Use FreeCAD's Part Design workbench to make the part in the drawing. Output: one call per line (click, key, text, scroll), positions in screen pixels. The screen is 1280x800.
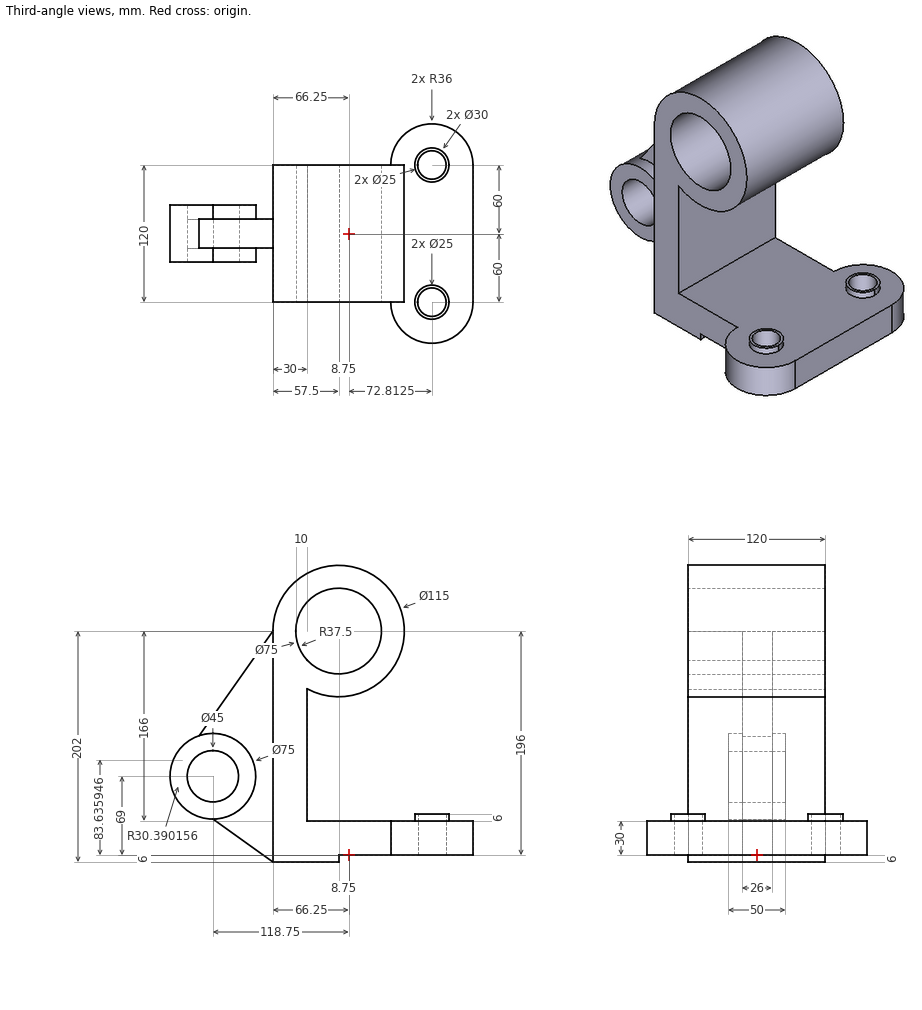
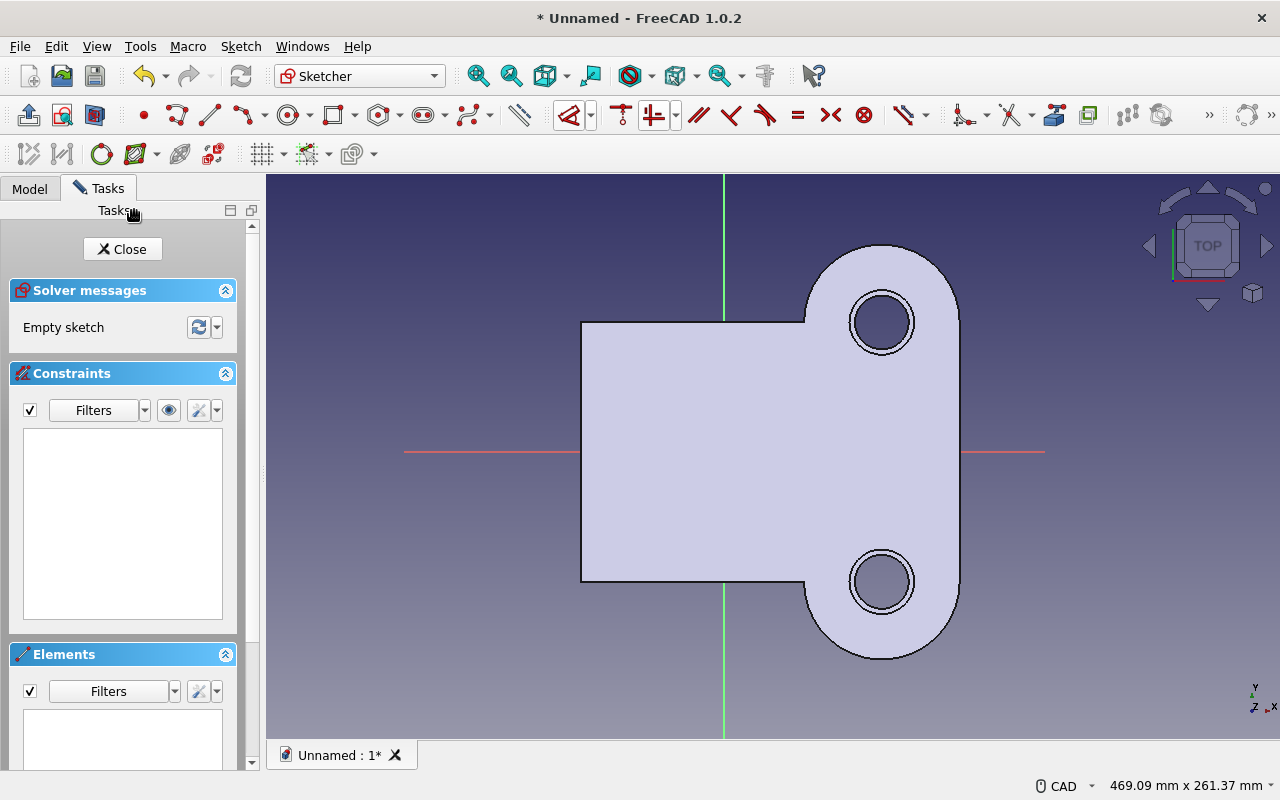
key(q)
key(s)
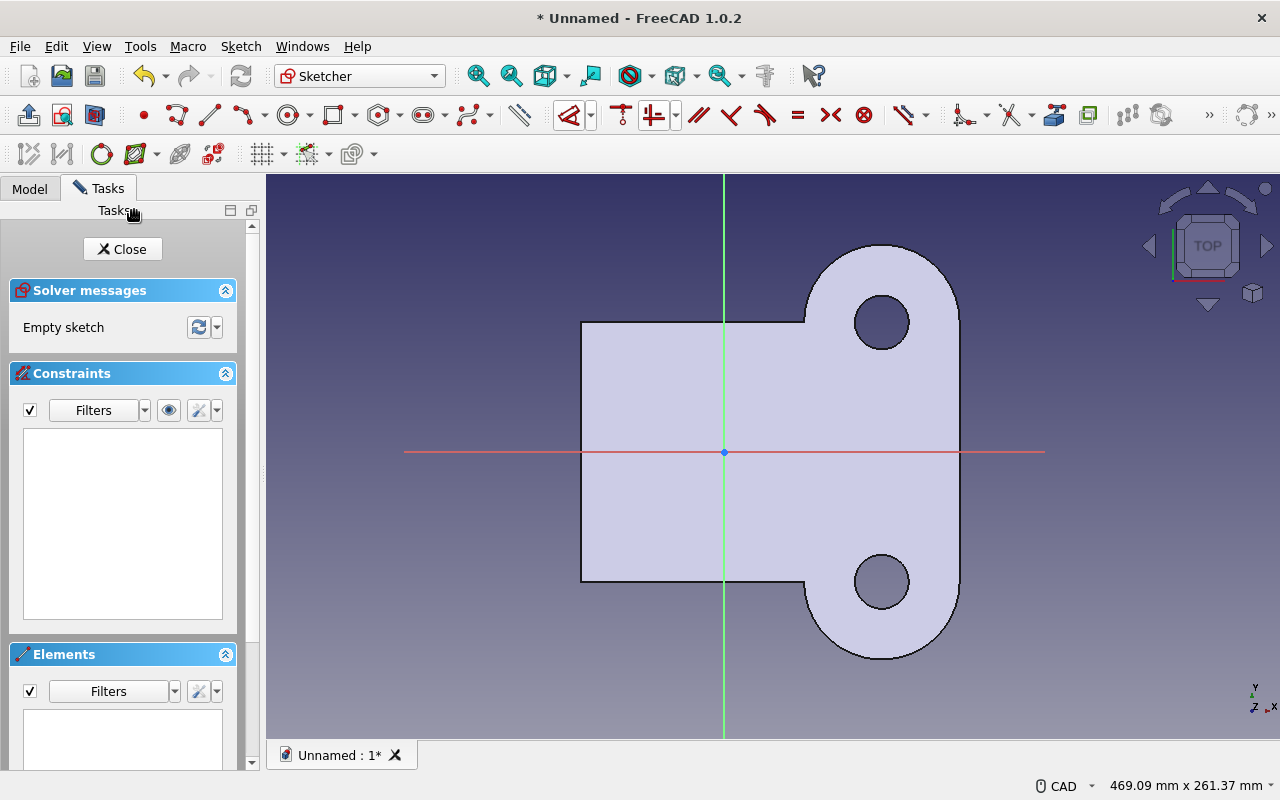
scroll(548, 443, up, 2)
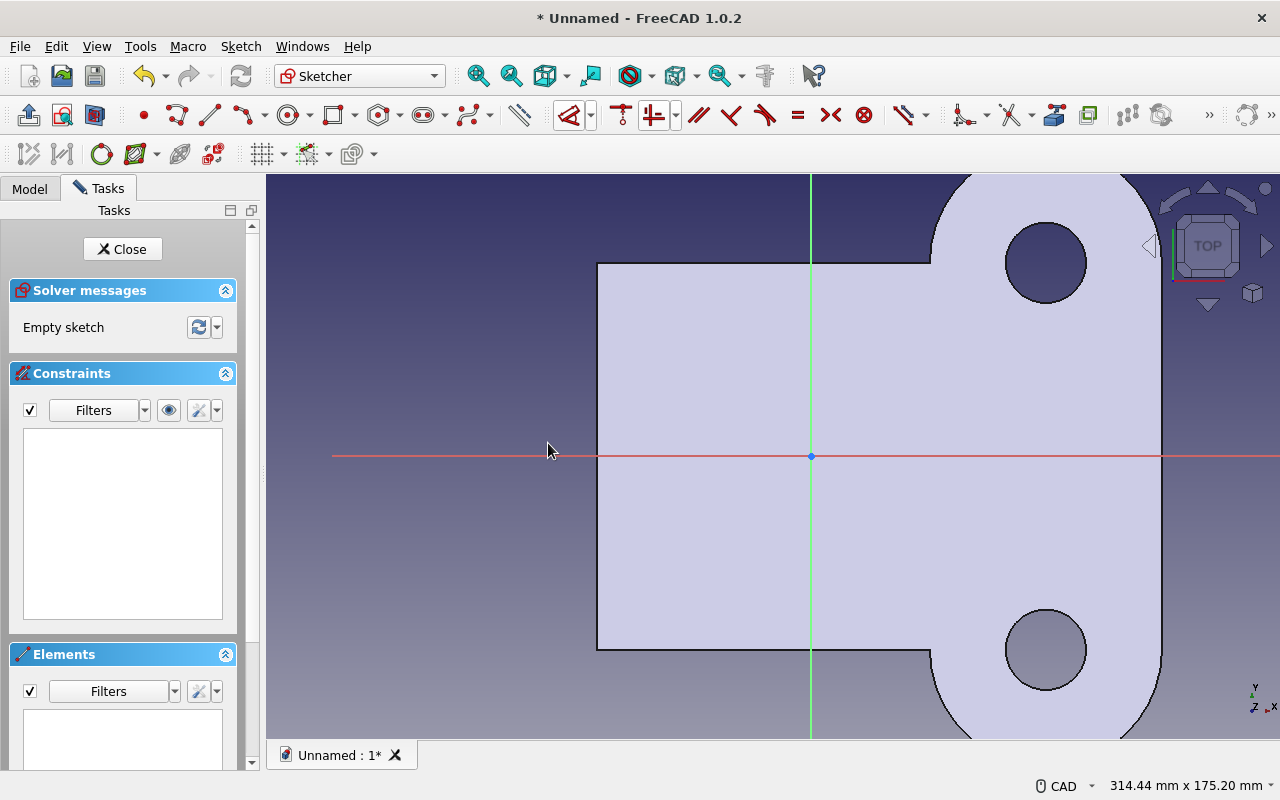
key(g)
key(r)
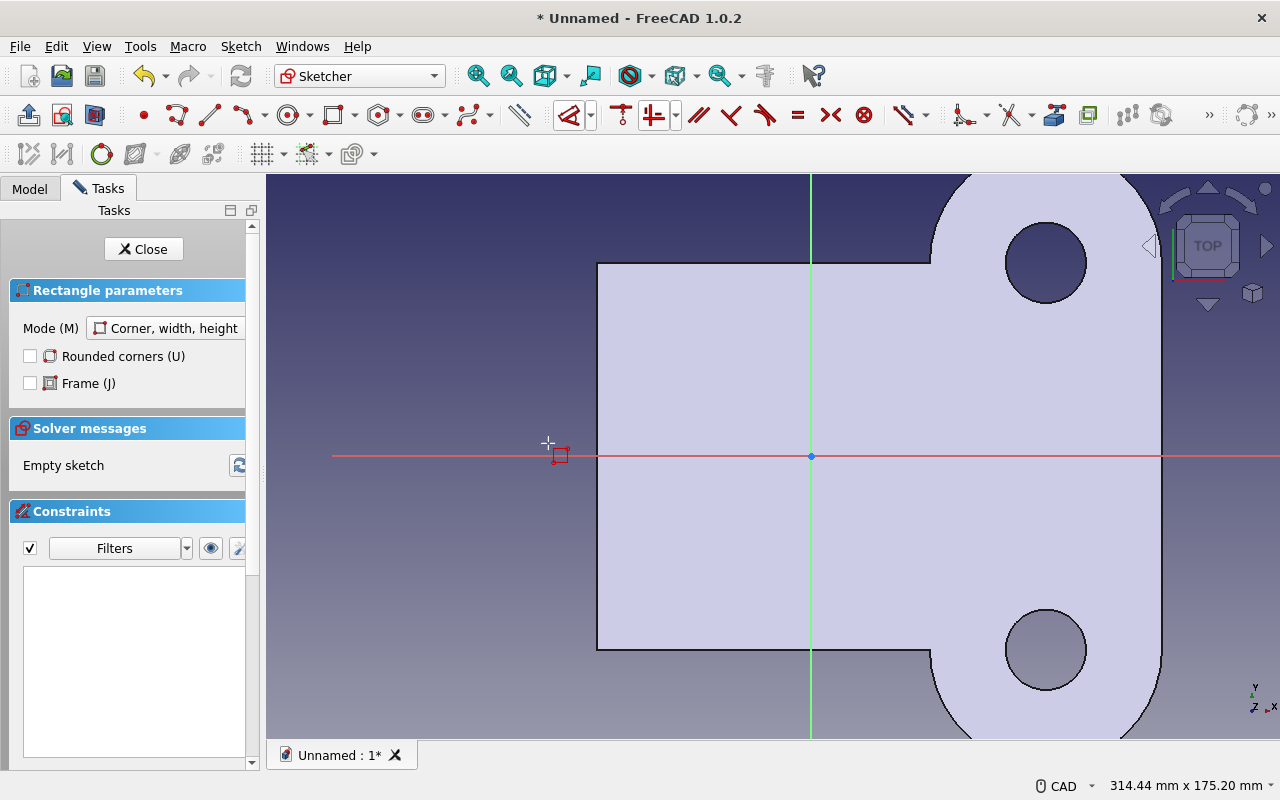
click(597, 263)
click(783, 650)
key(Escape)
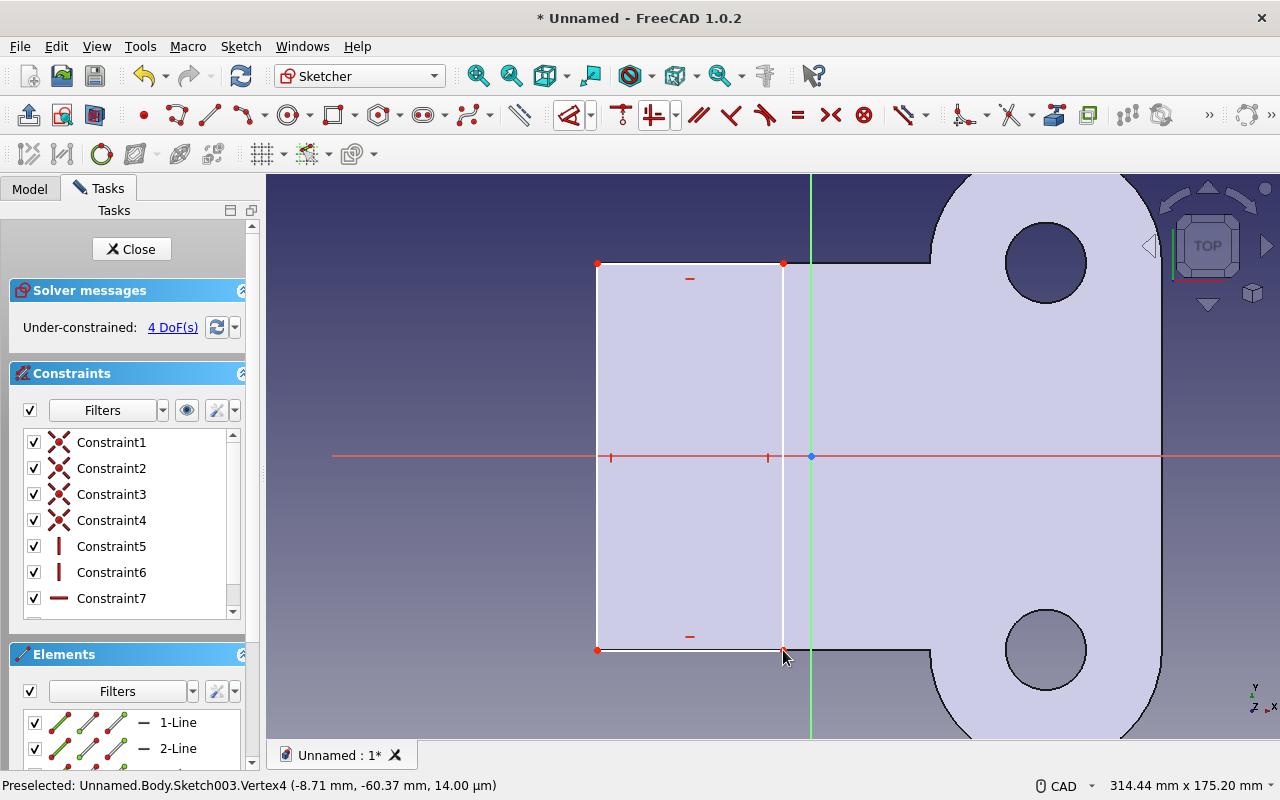
click(597, 380)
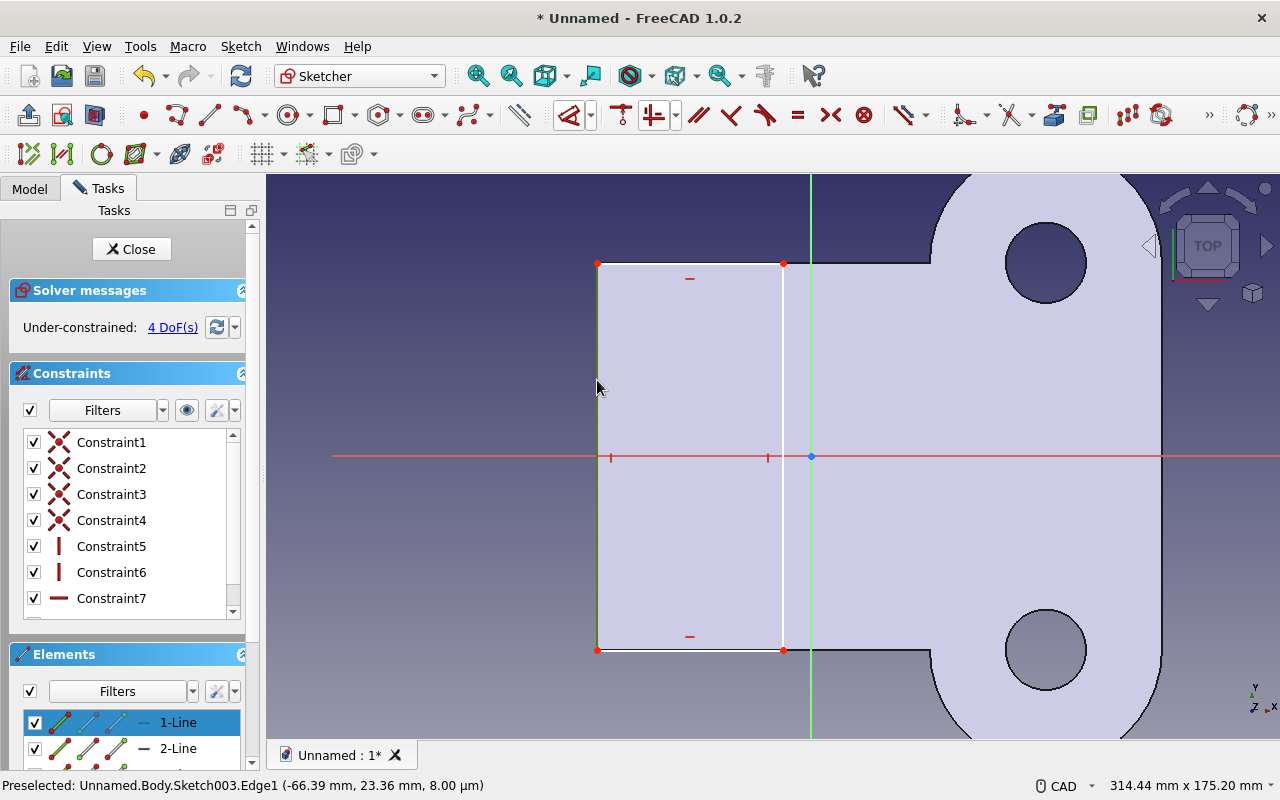
key(i)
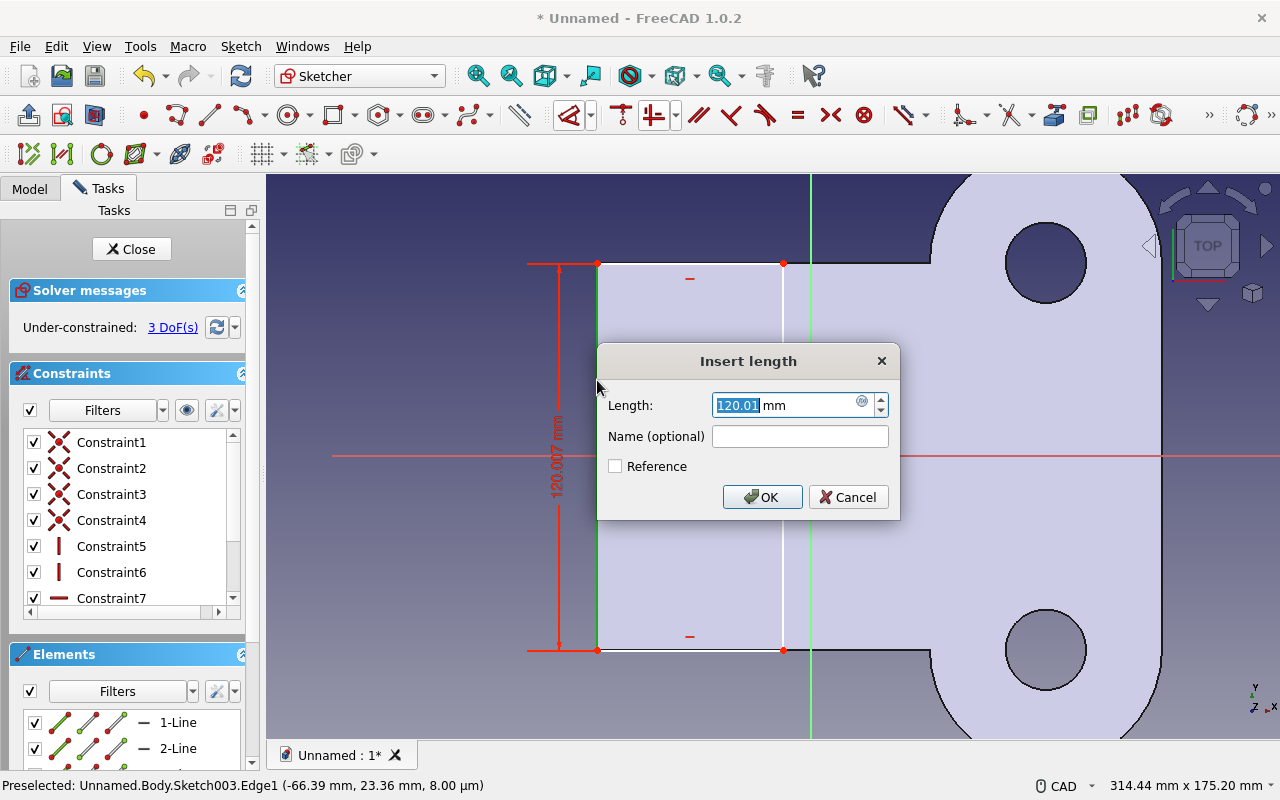
text(120)
key(Return)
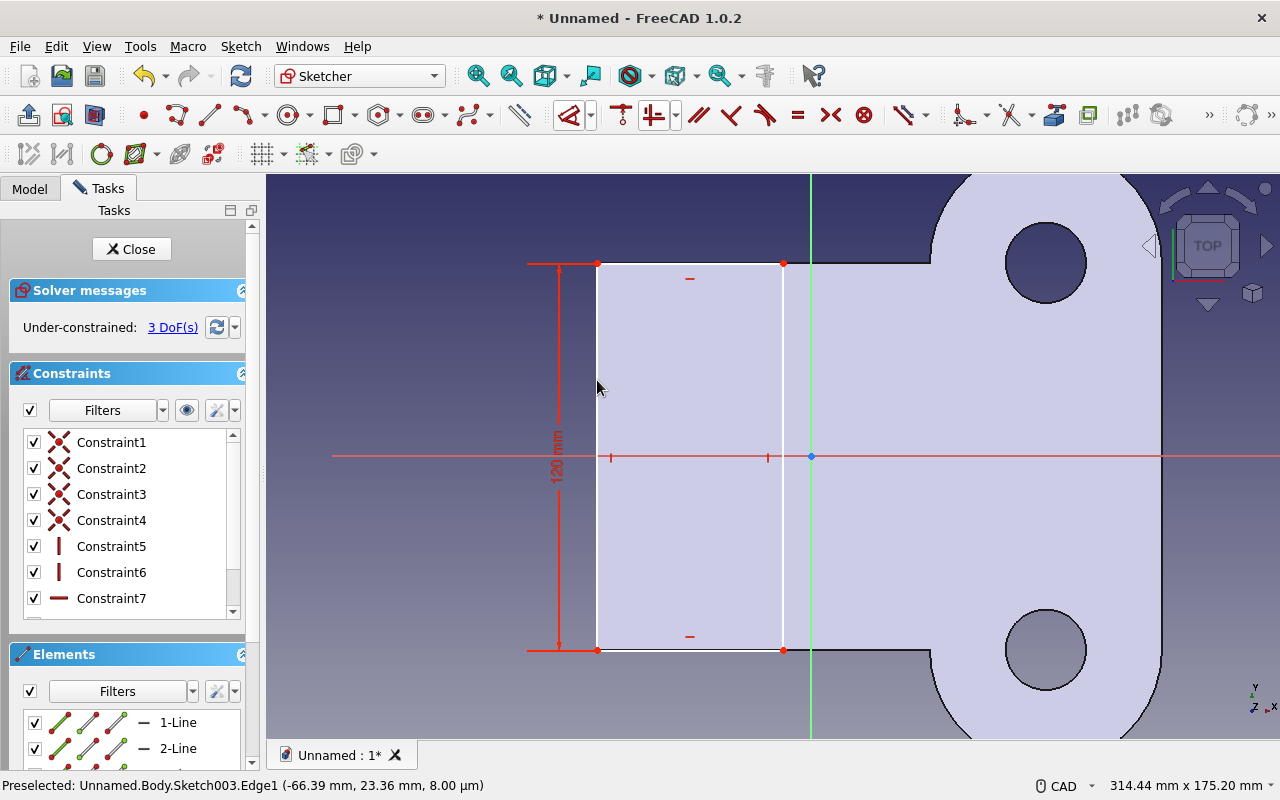
click(597, 264)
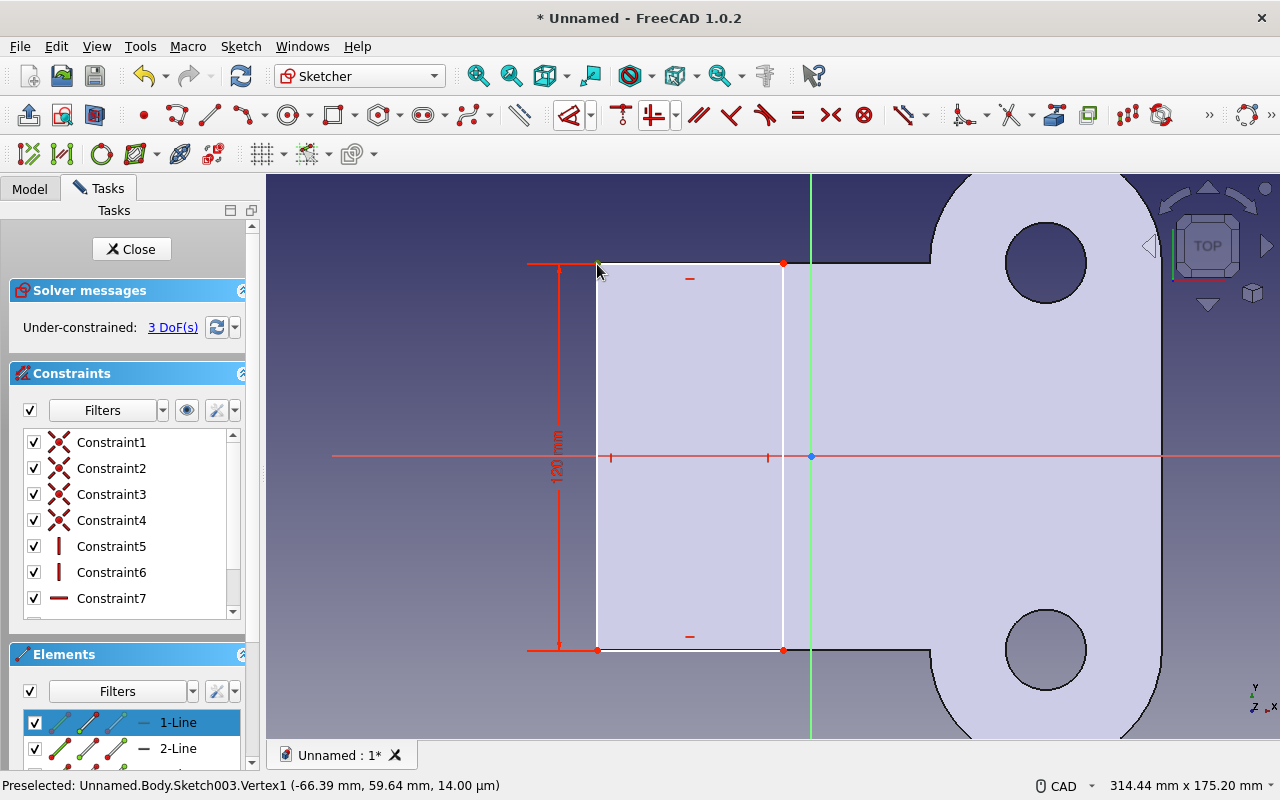
key(i)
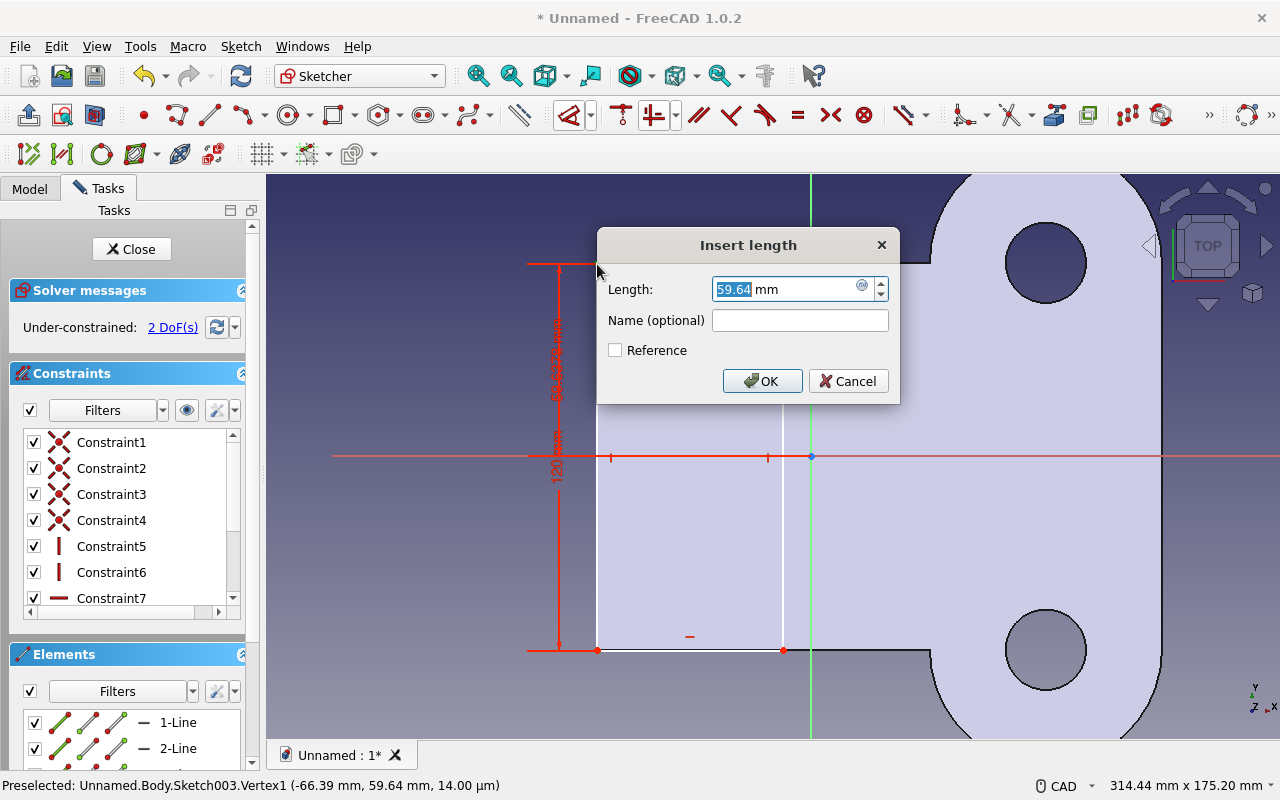
text(60)
key(Return)